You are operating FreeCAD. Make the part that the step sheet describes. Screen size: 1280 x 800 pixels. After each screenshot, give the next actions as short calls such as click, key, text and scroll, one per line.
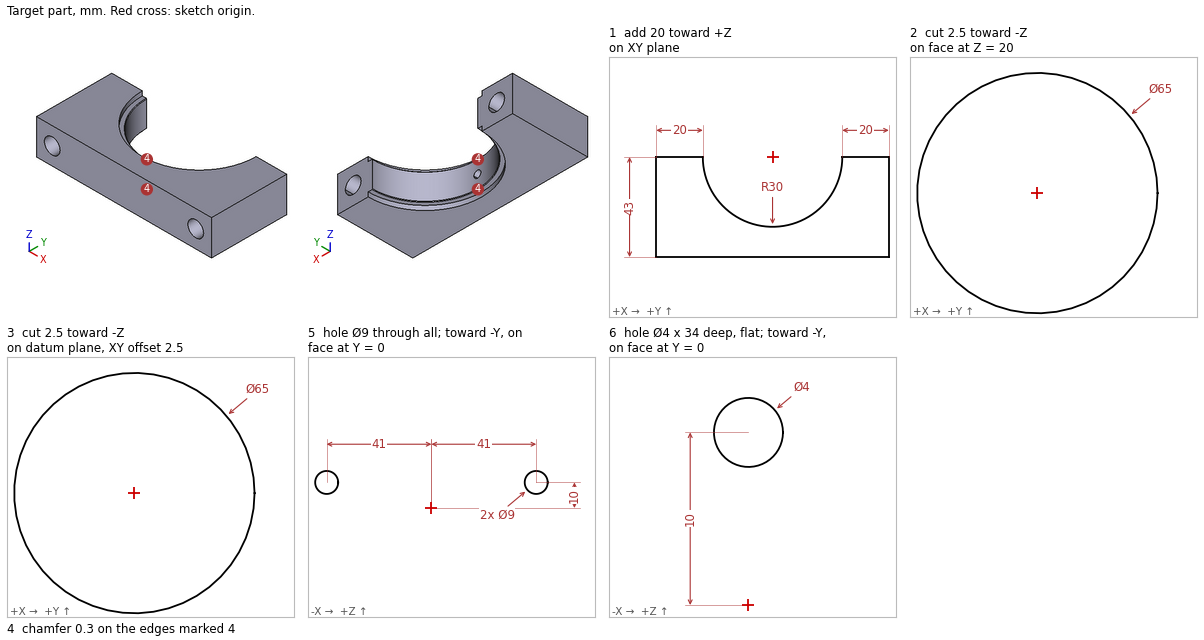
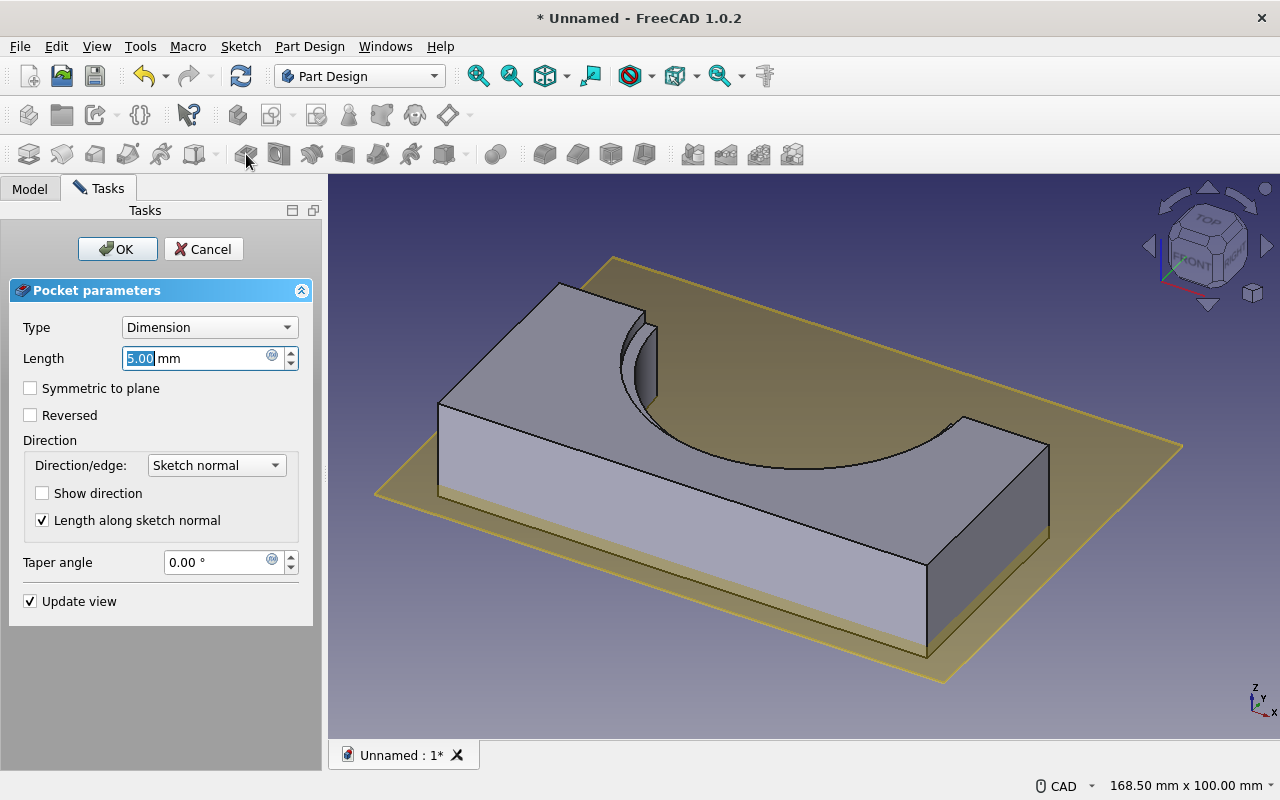
text(2.5)
key(Tab)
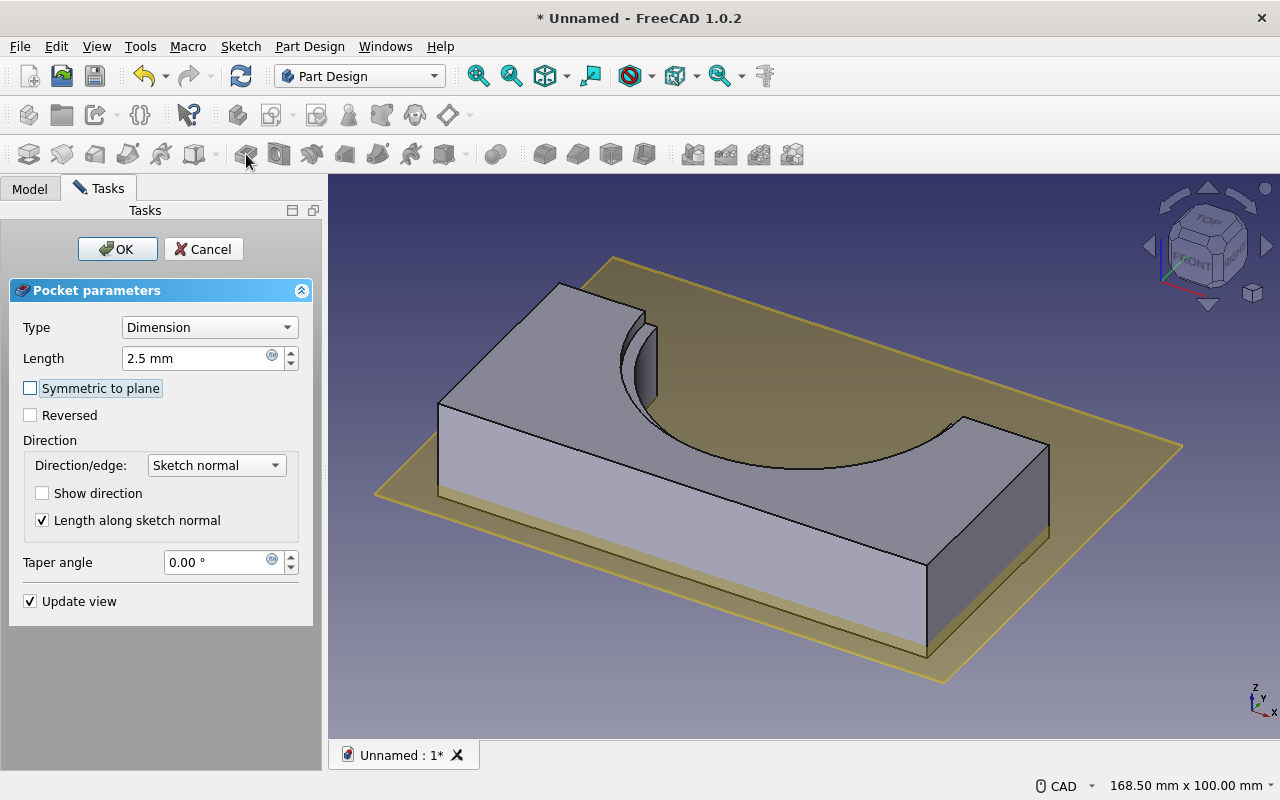
click(118, 249)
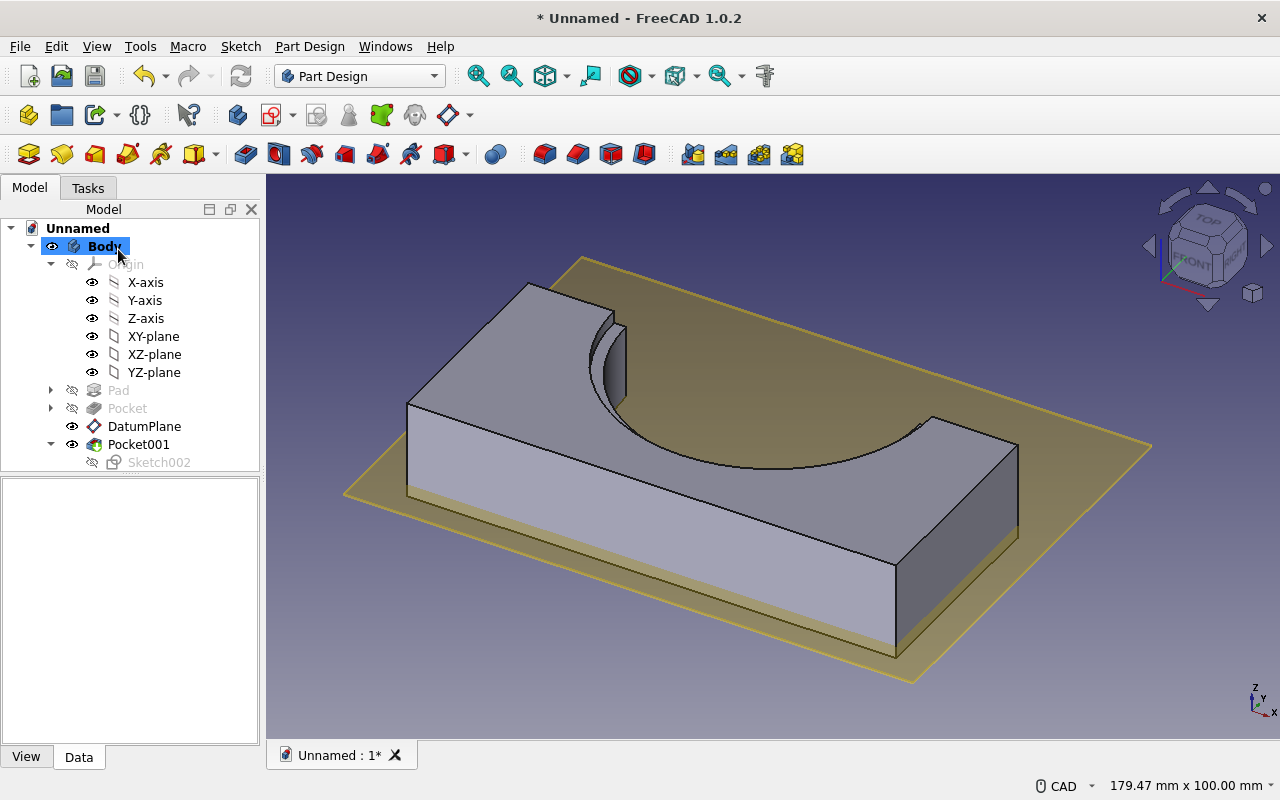
click(117, 426)
key(space)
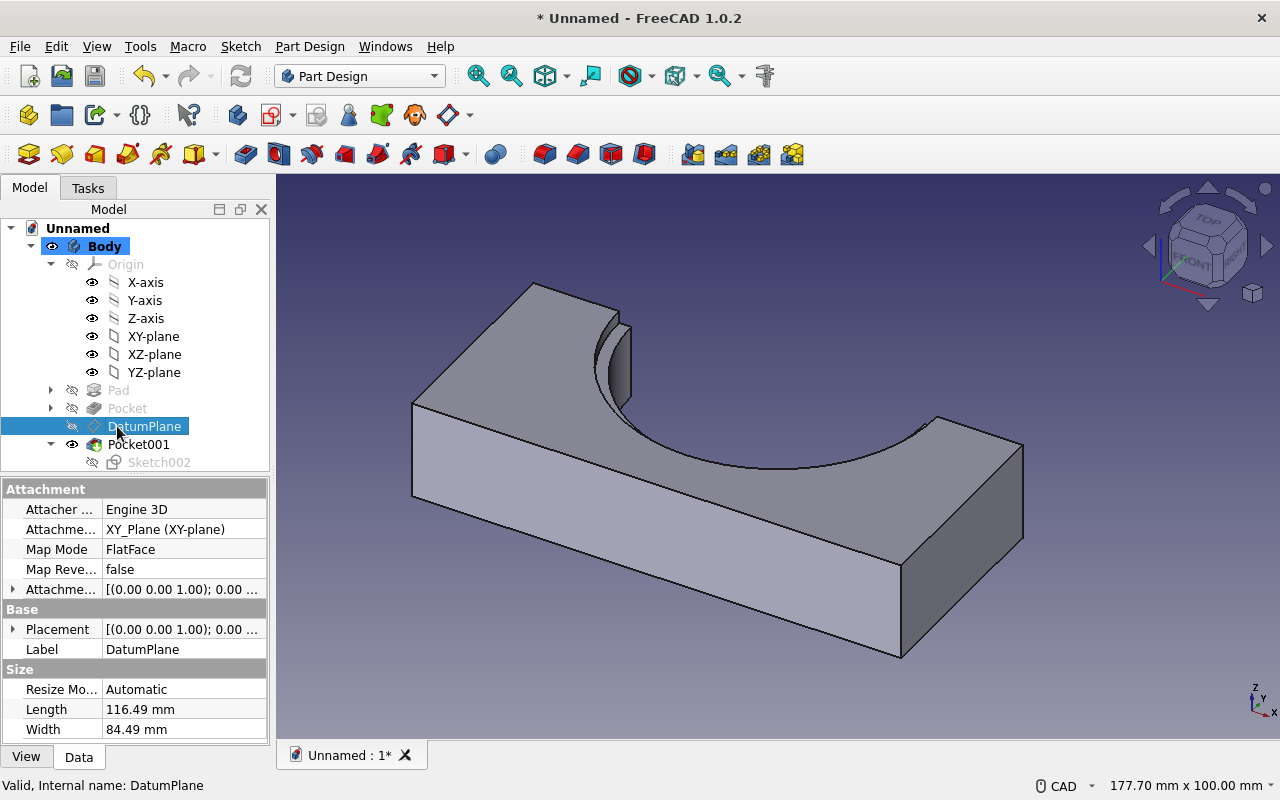
click(610, 360)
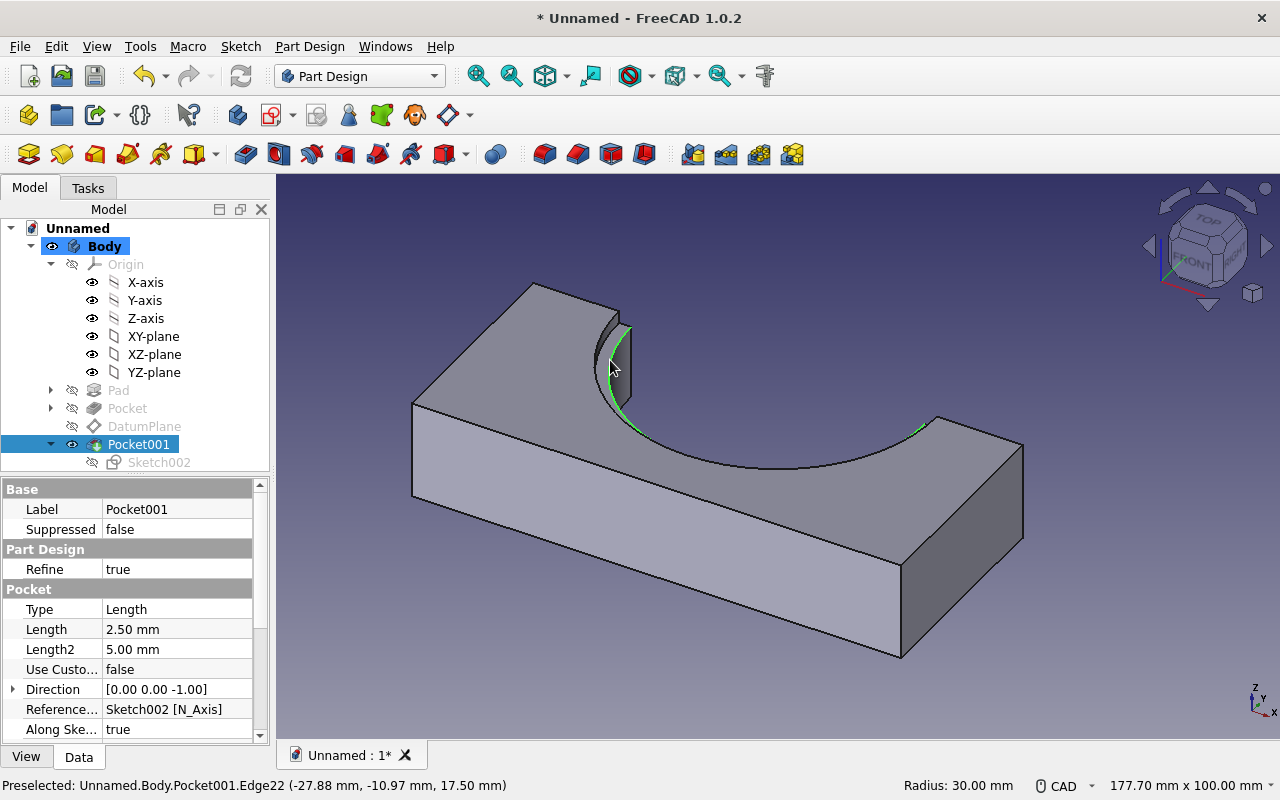
key(0)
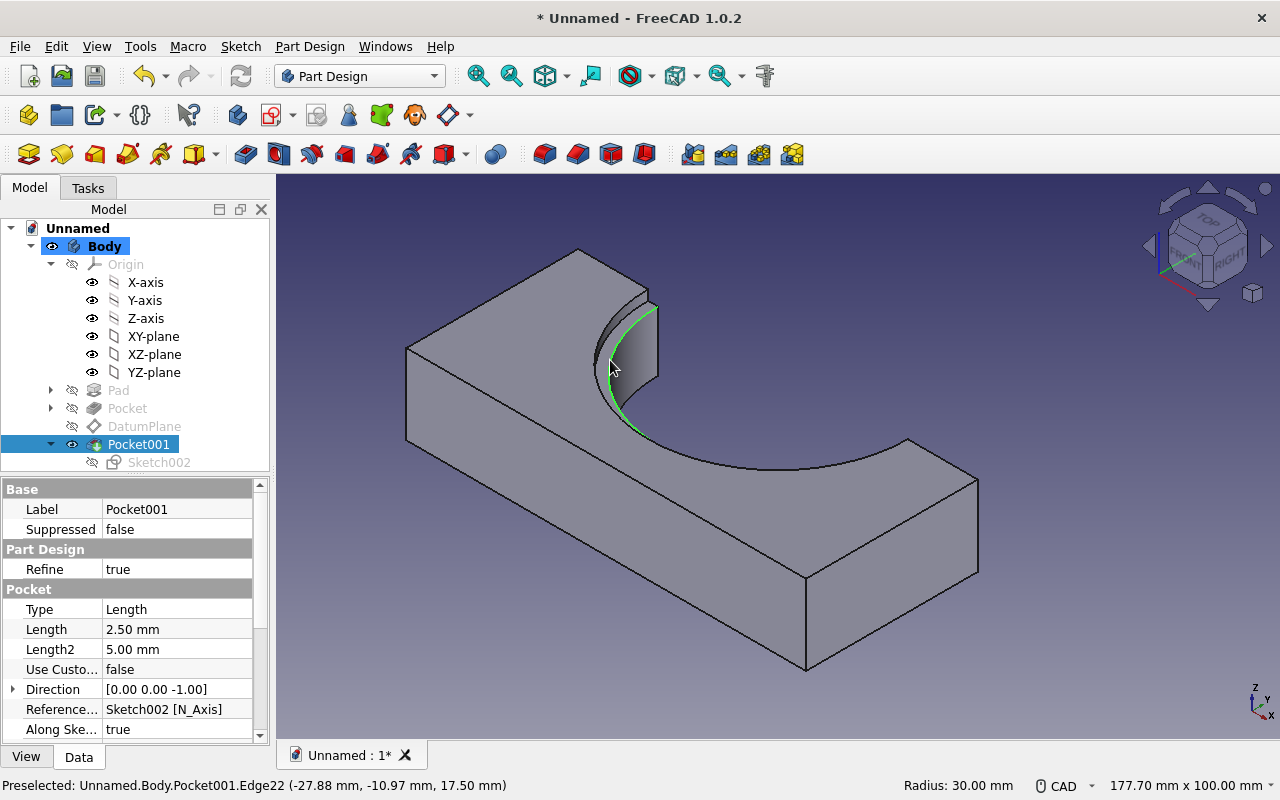
key(2)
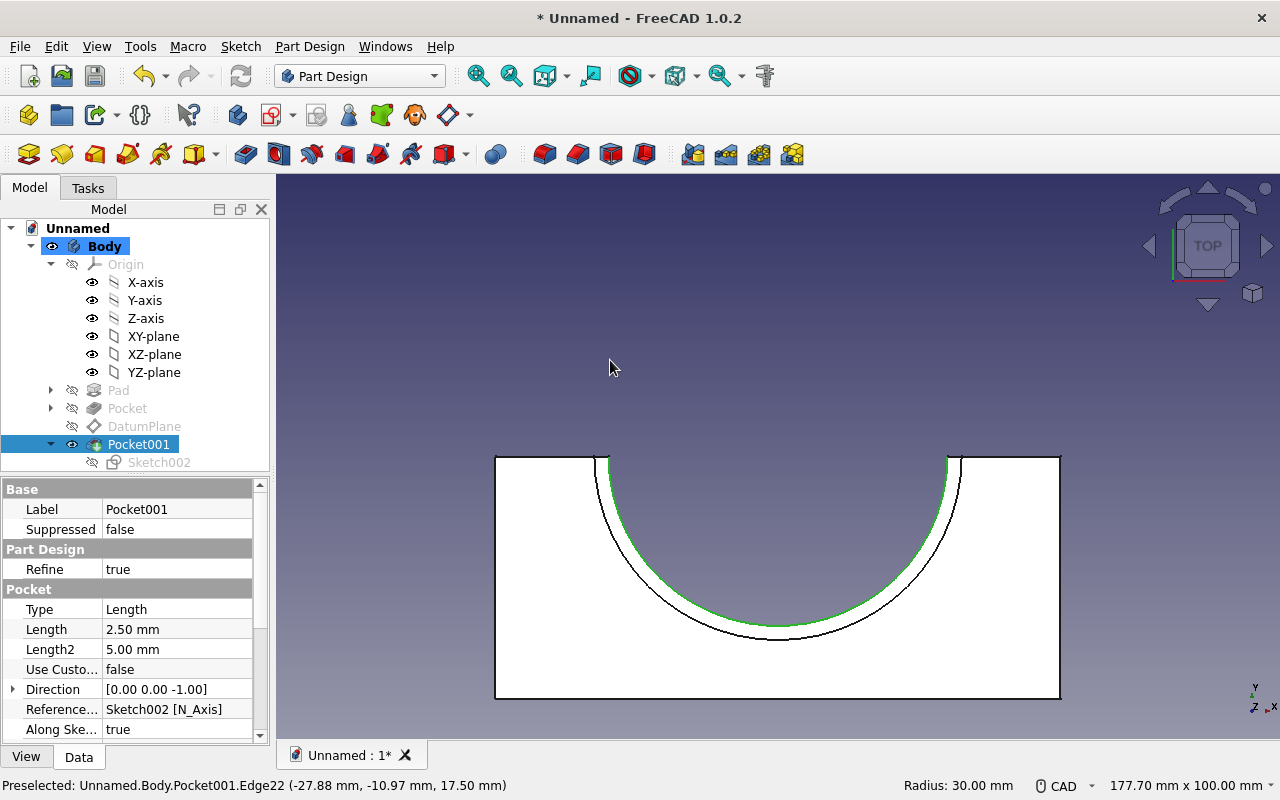
key(1)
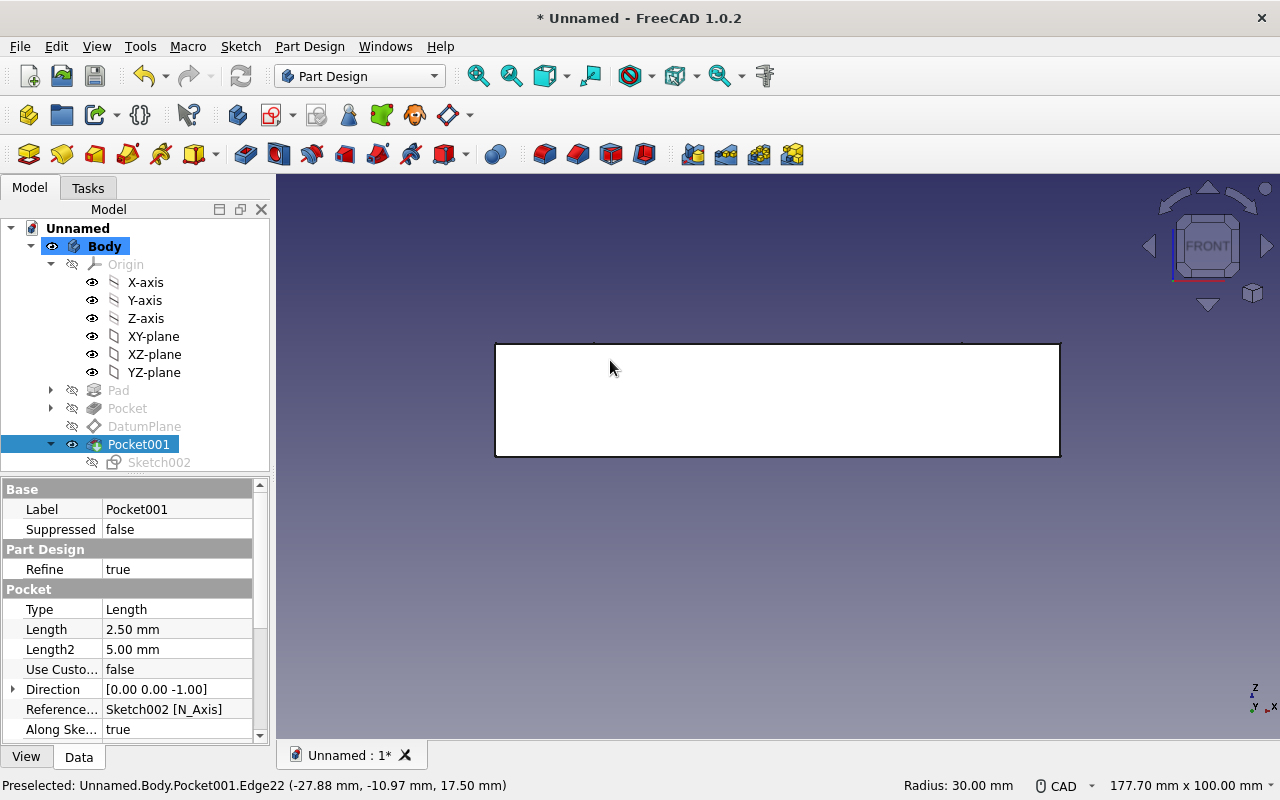
key(3)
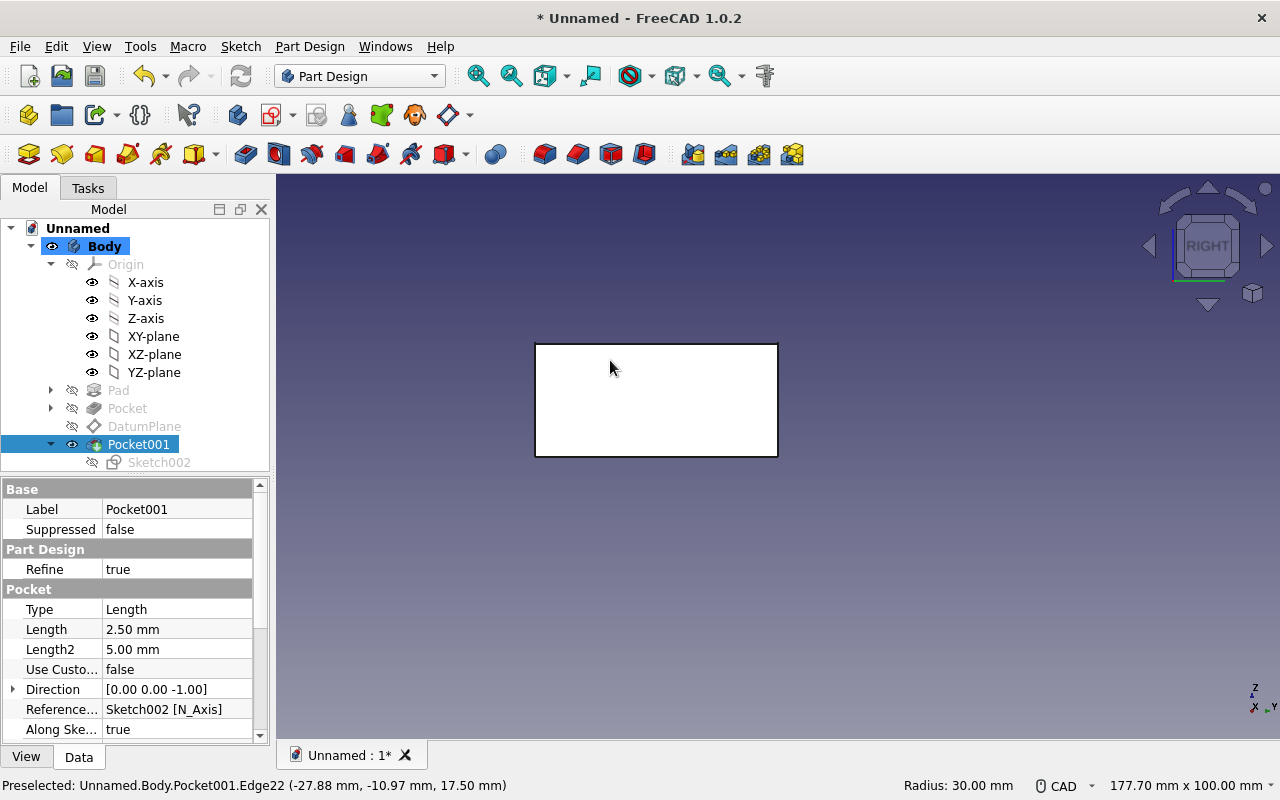
click(479, 76)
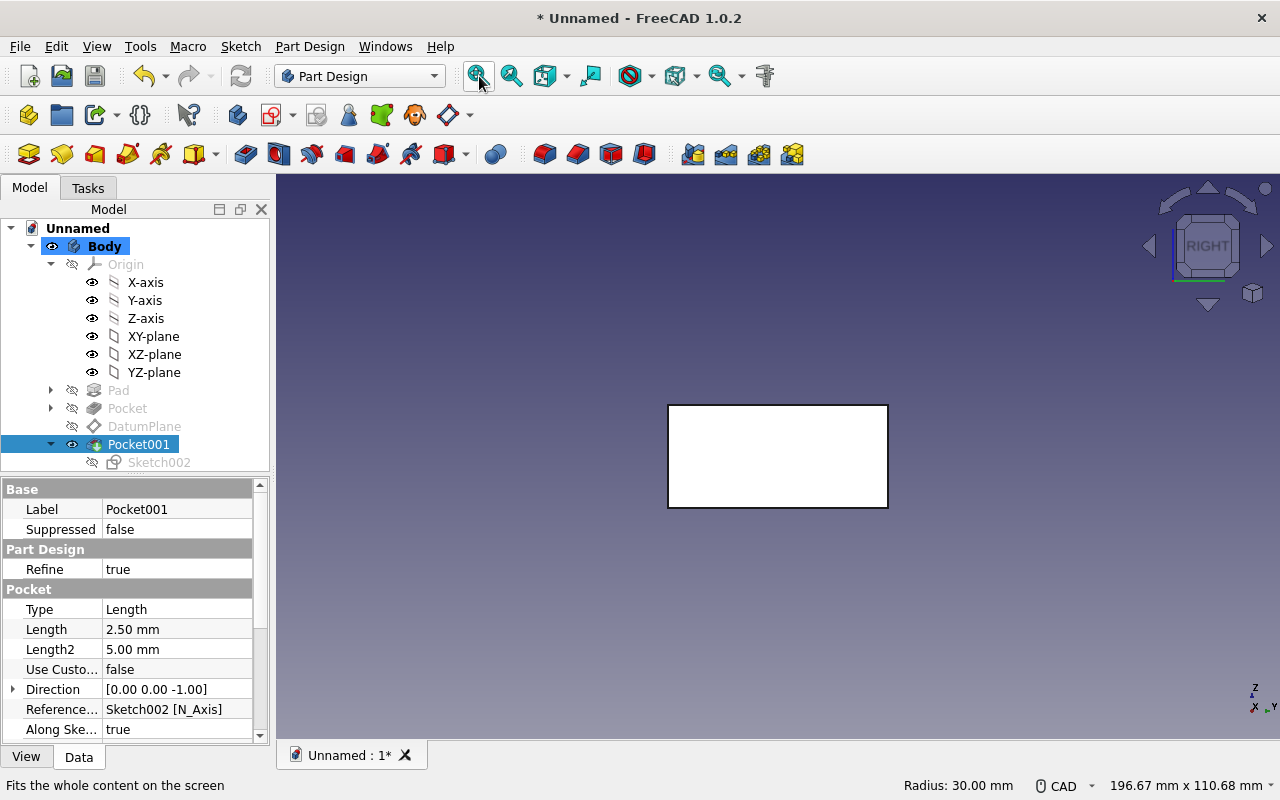
key(5)